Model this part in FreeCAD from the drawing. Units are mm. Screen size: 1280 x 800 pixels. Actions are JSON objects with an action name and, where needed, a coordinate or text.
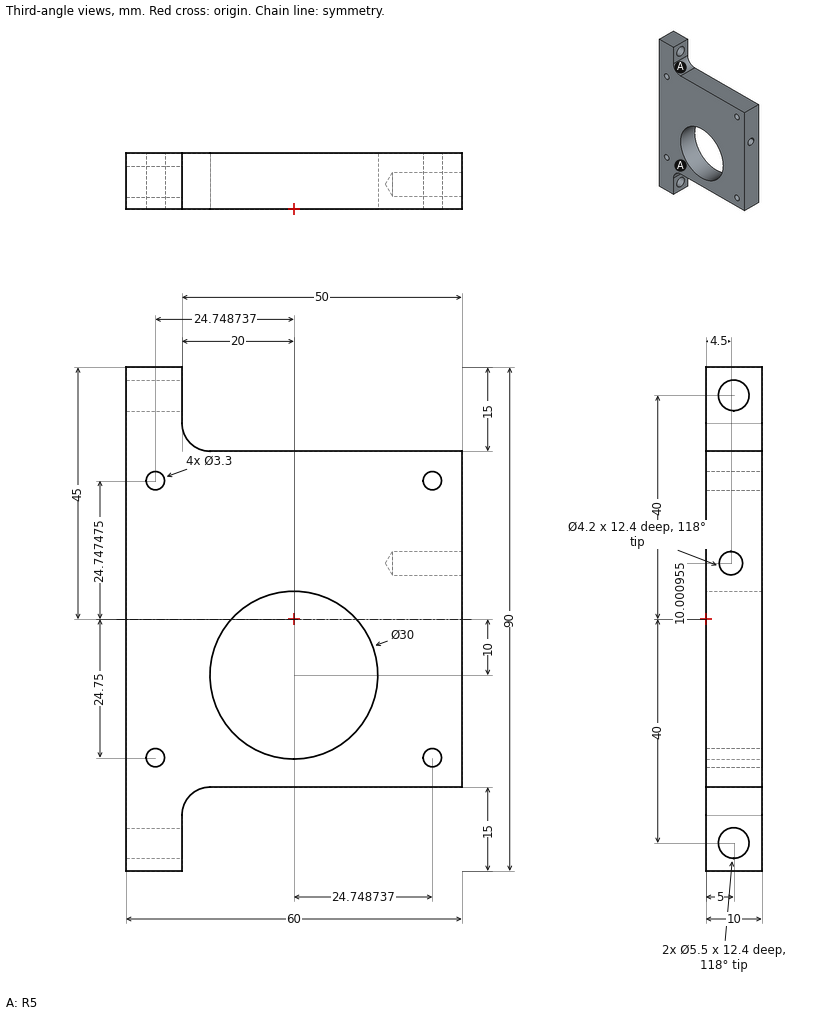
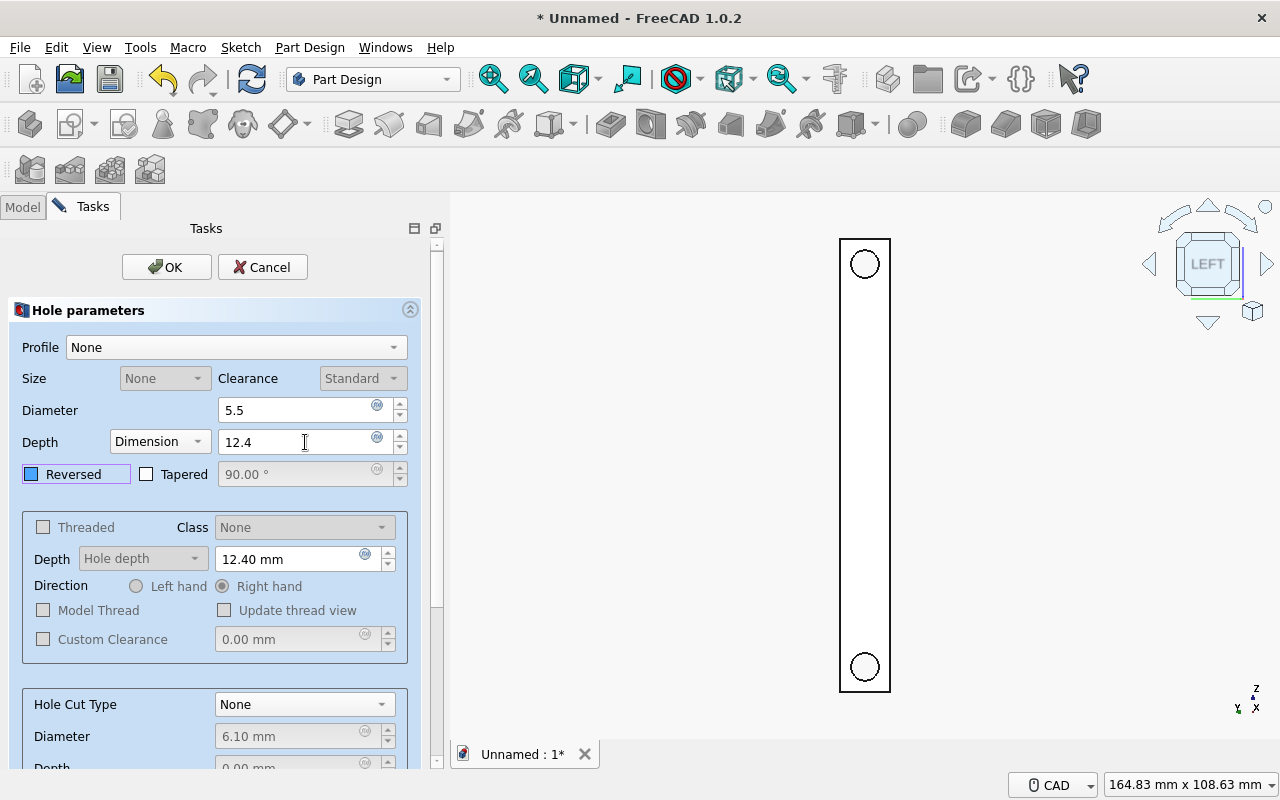
{"action": "left_click", "coordinate": [167, 267]}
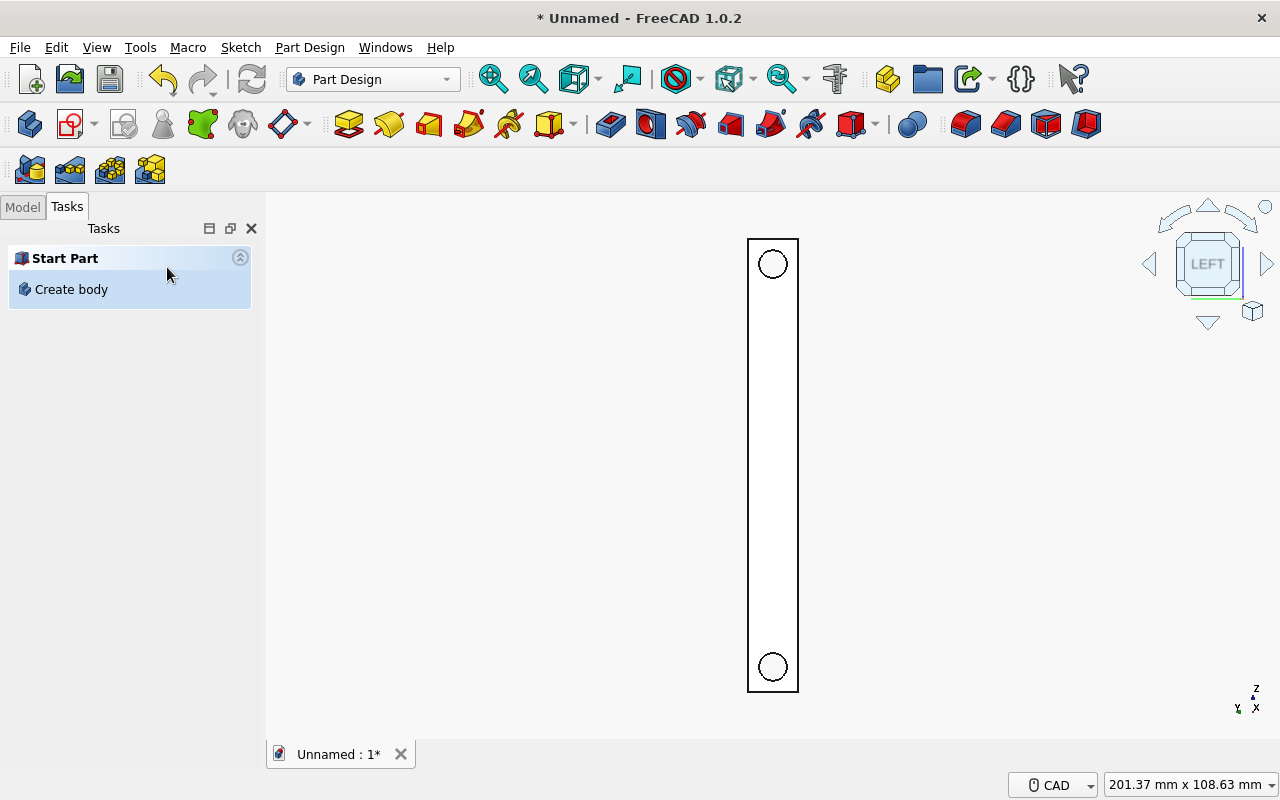
{"action": "key", "text": "0"}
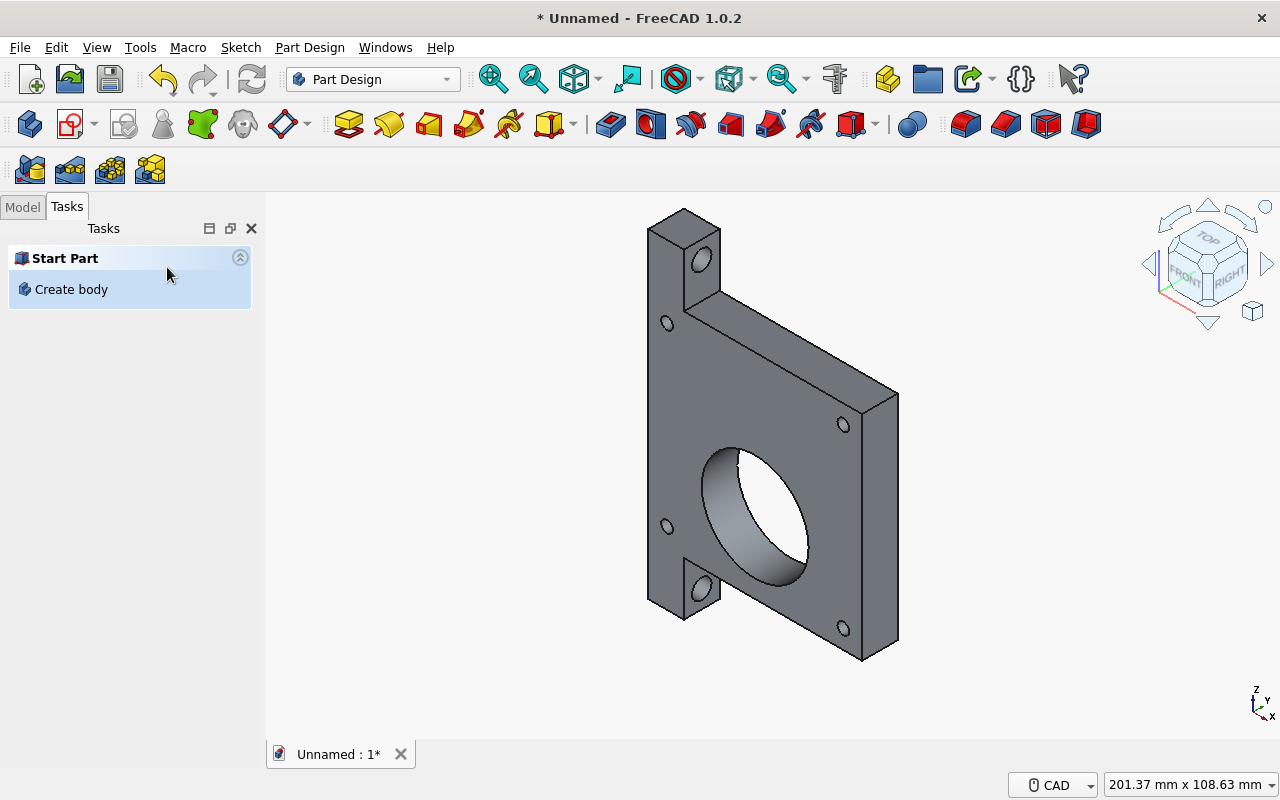
{"action": "key", "text": "2"}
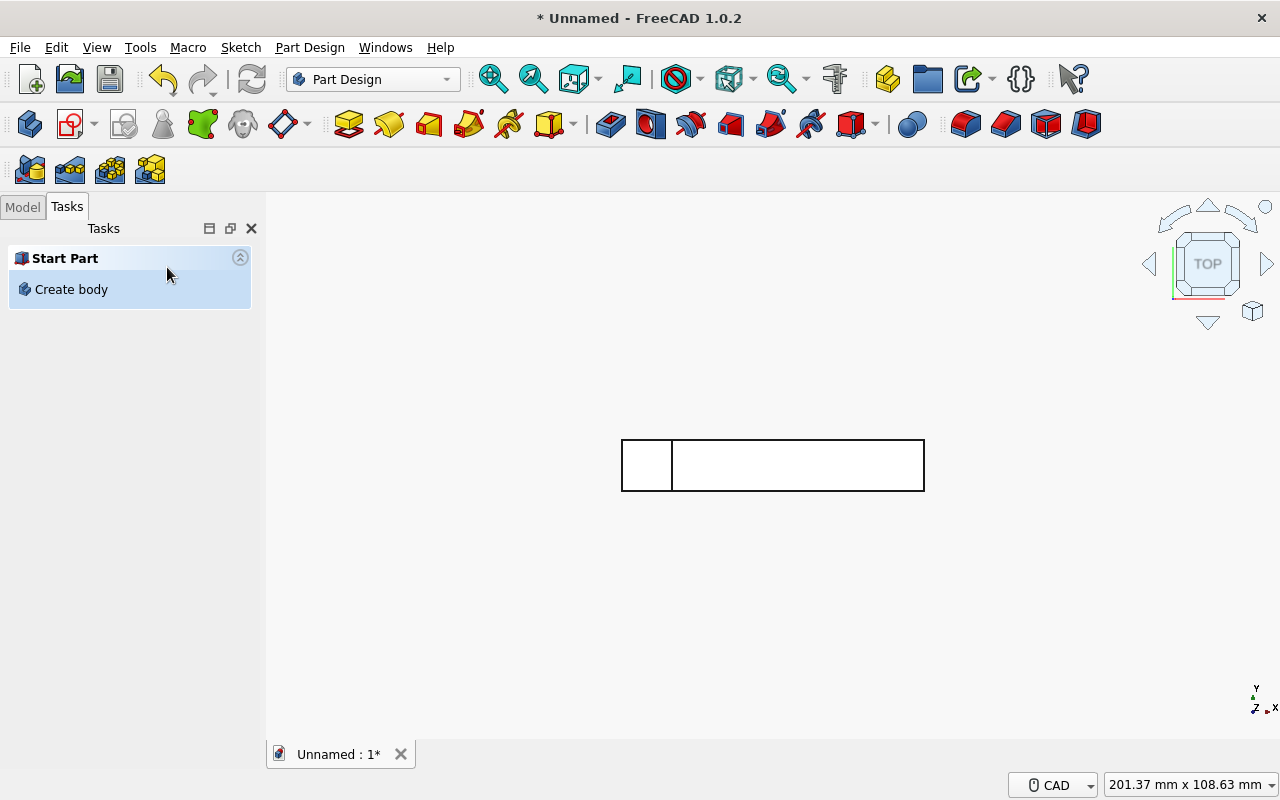
{"action": "key", "text": "v f"}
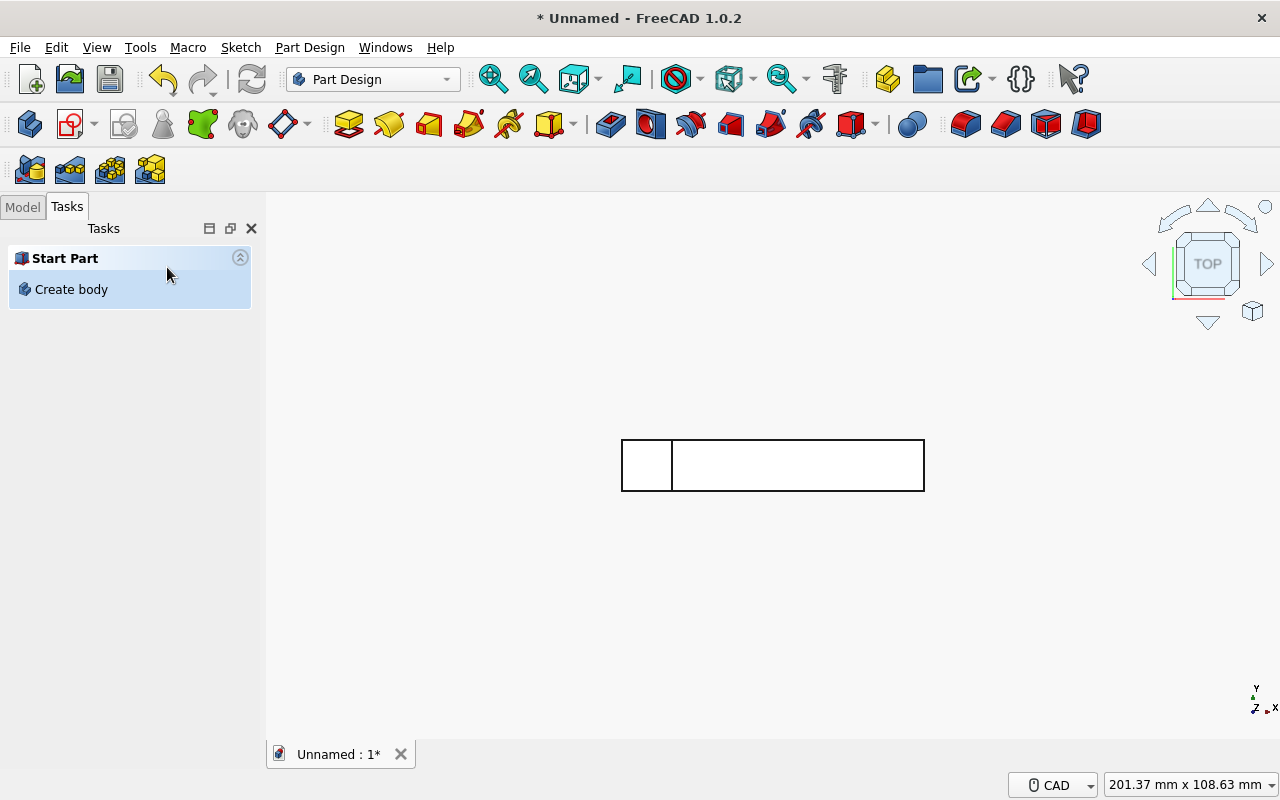
{"action": "key", "text": "1"}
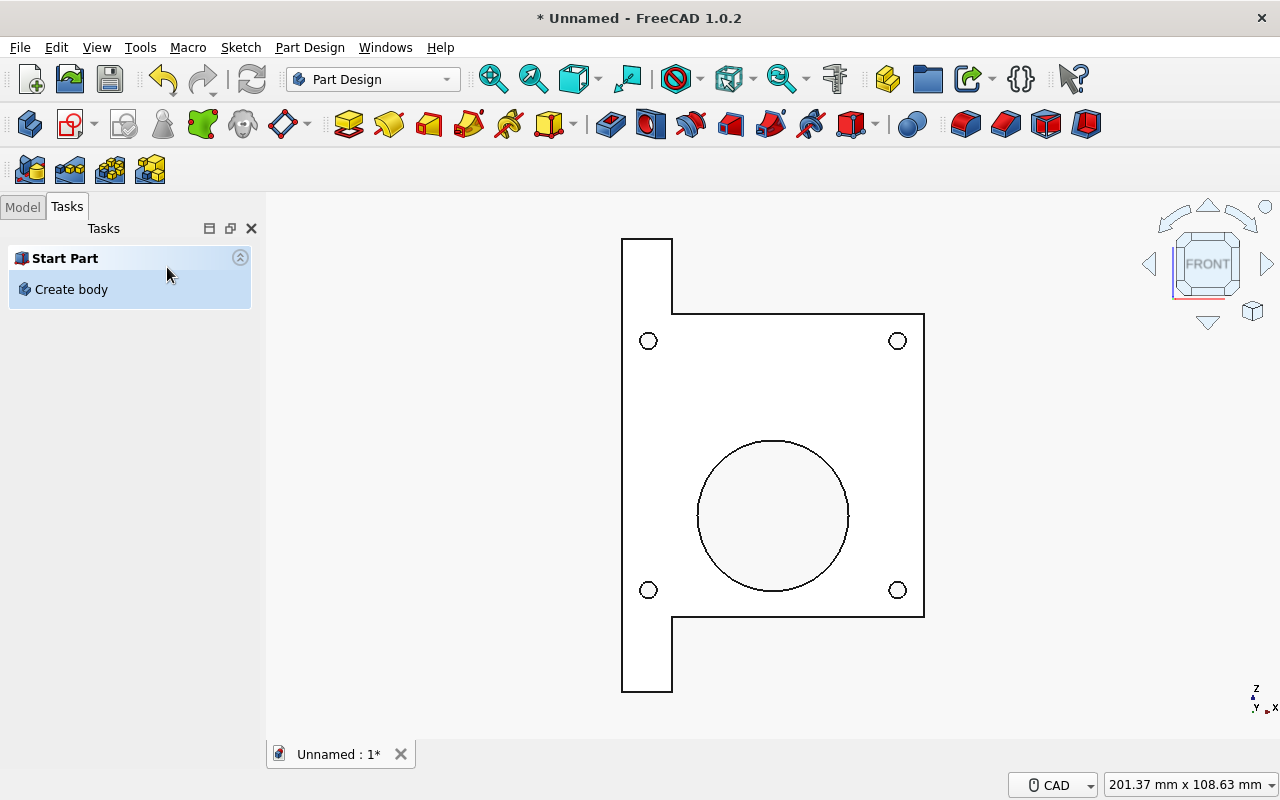
{"action": "key", "text": "3"}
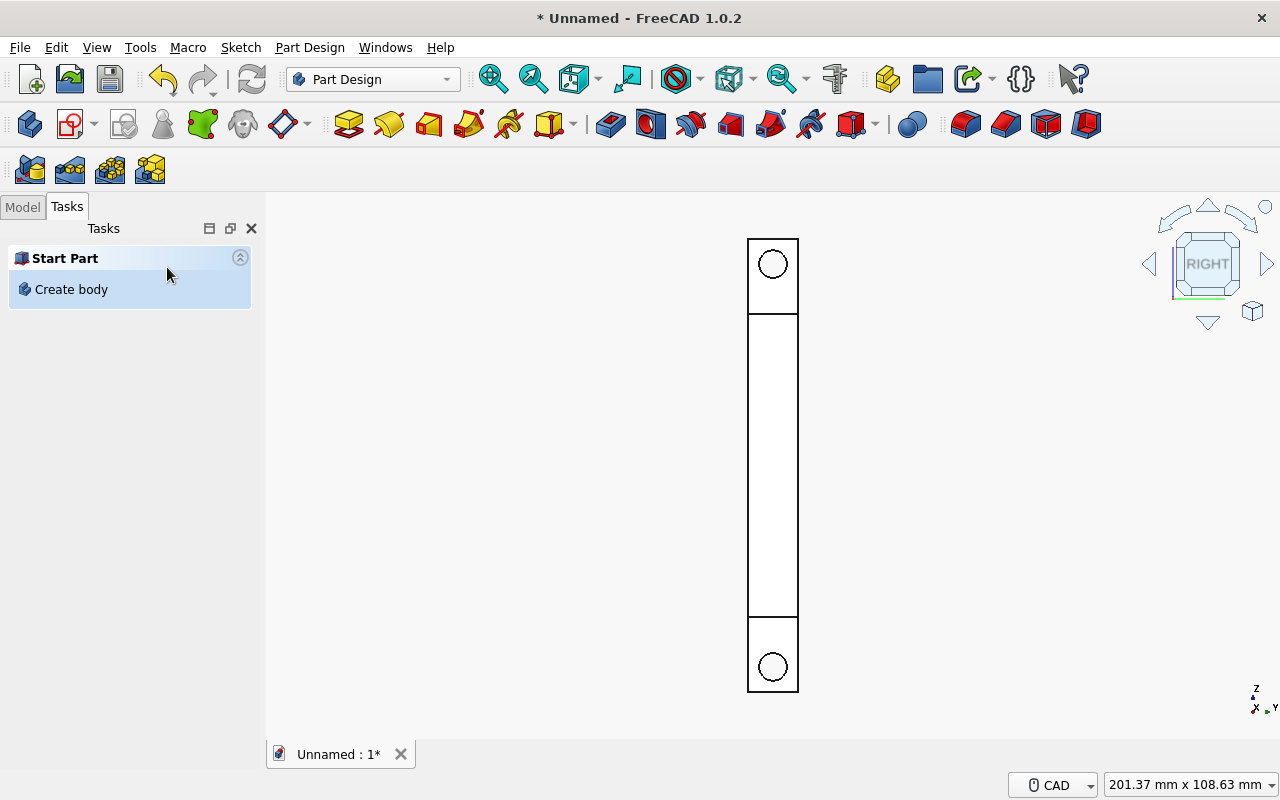
{"action": "key", "text": "5"}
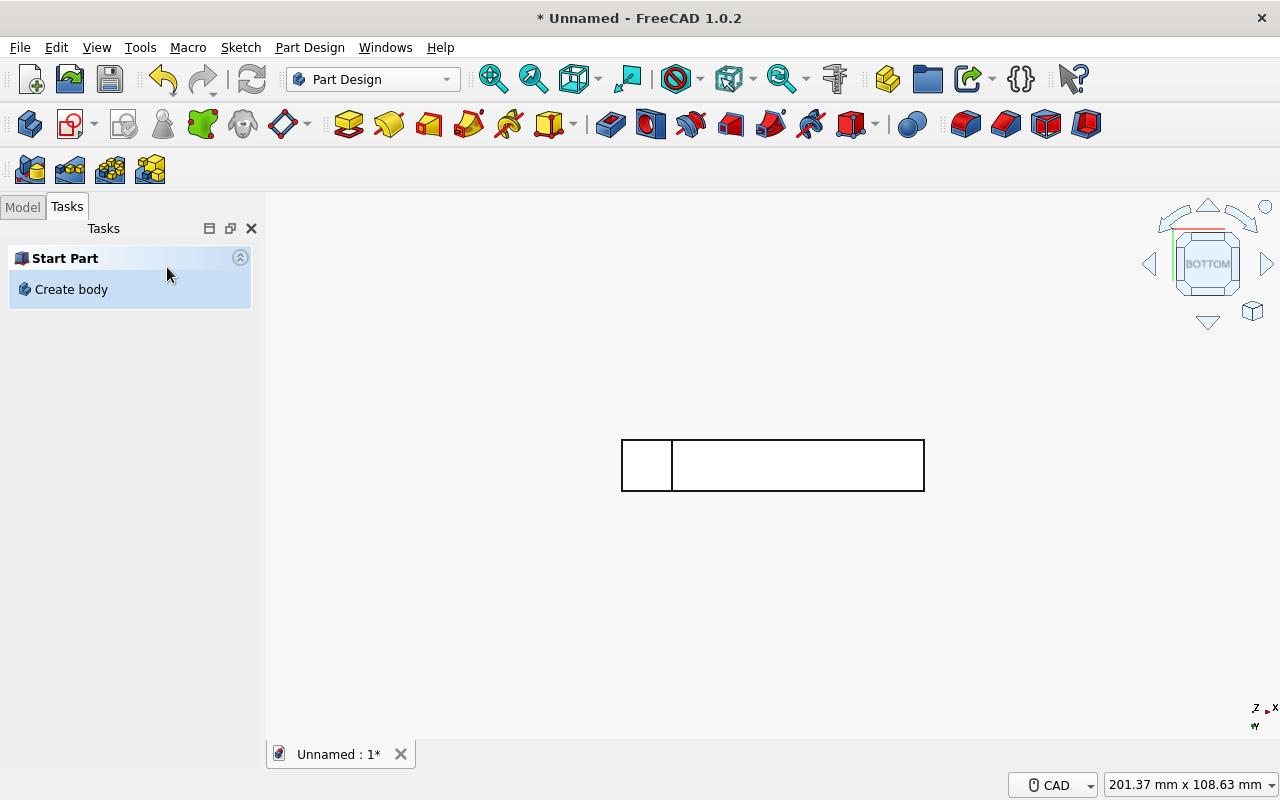
{"action": "key", "text": "v f"}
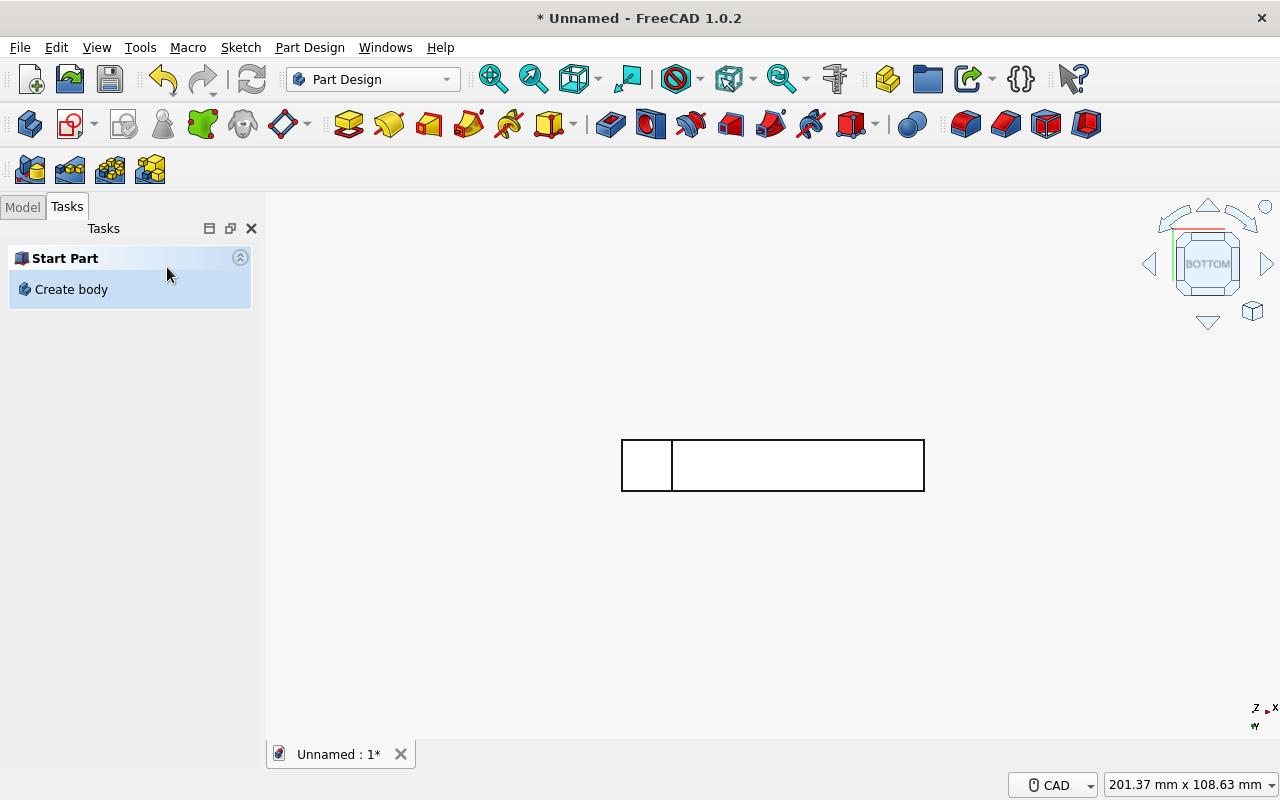
{"action": "key", "text": "4"}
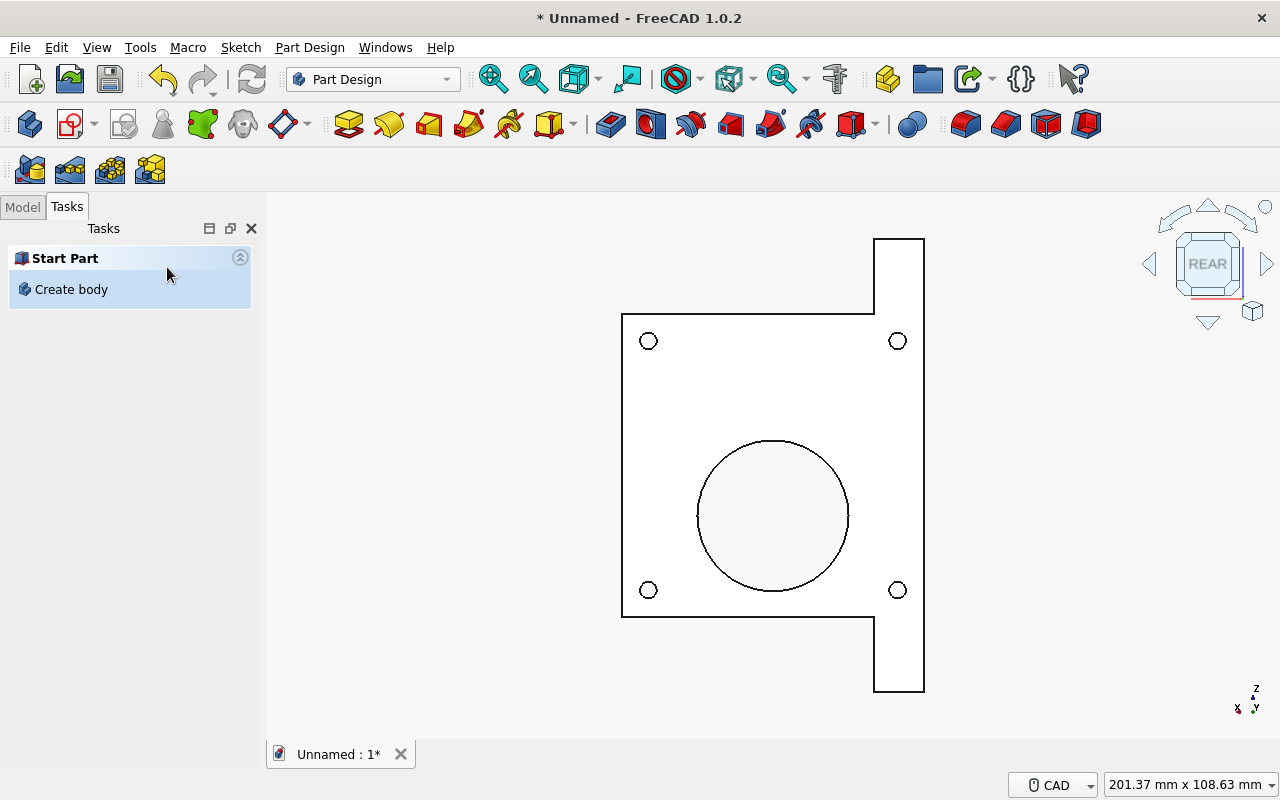
{"action": "key", "text": "6"}